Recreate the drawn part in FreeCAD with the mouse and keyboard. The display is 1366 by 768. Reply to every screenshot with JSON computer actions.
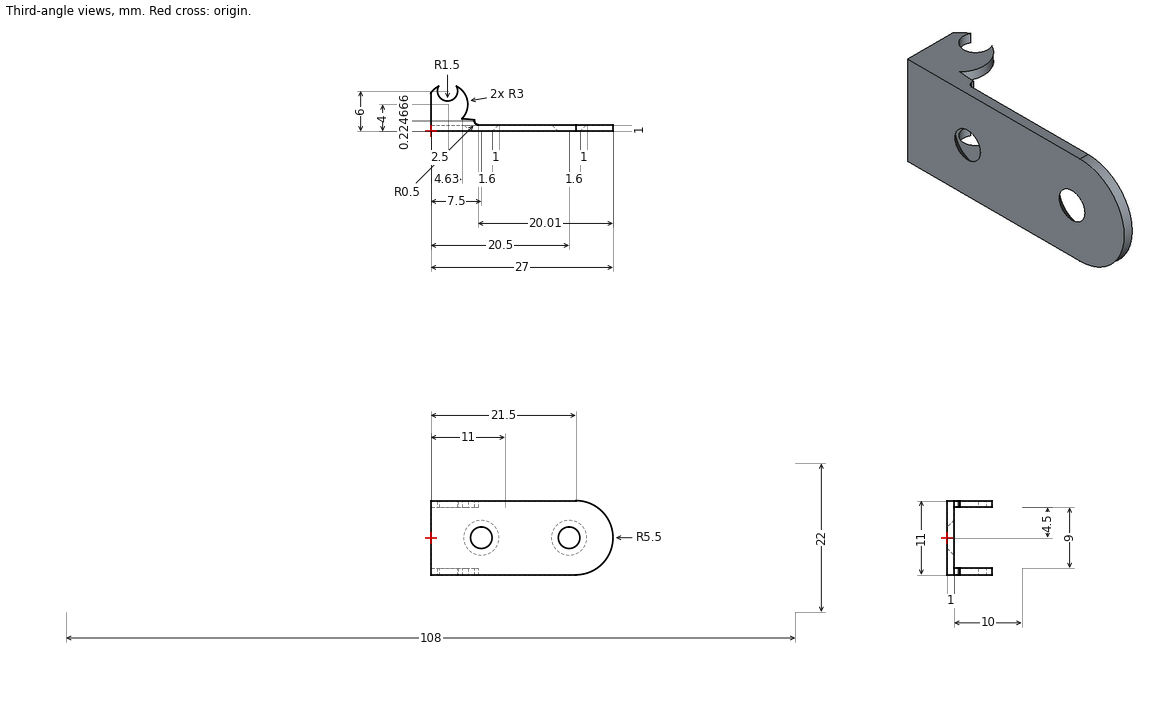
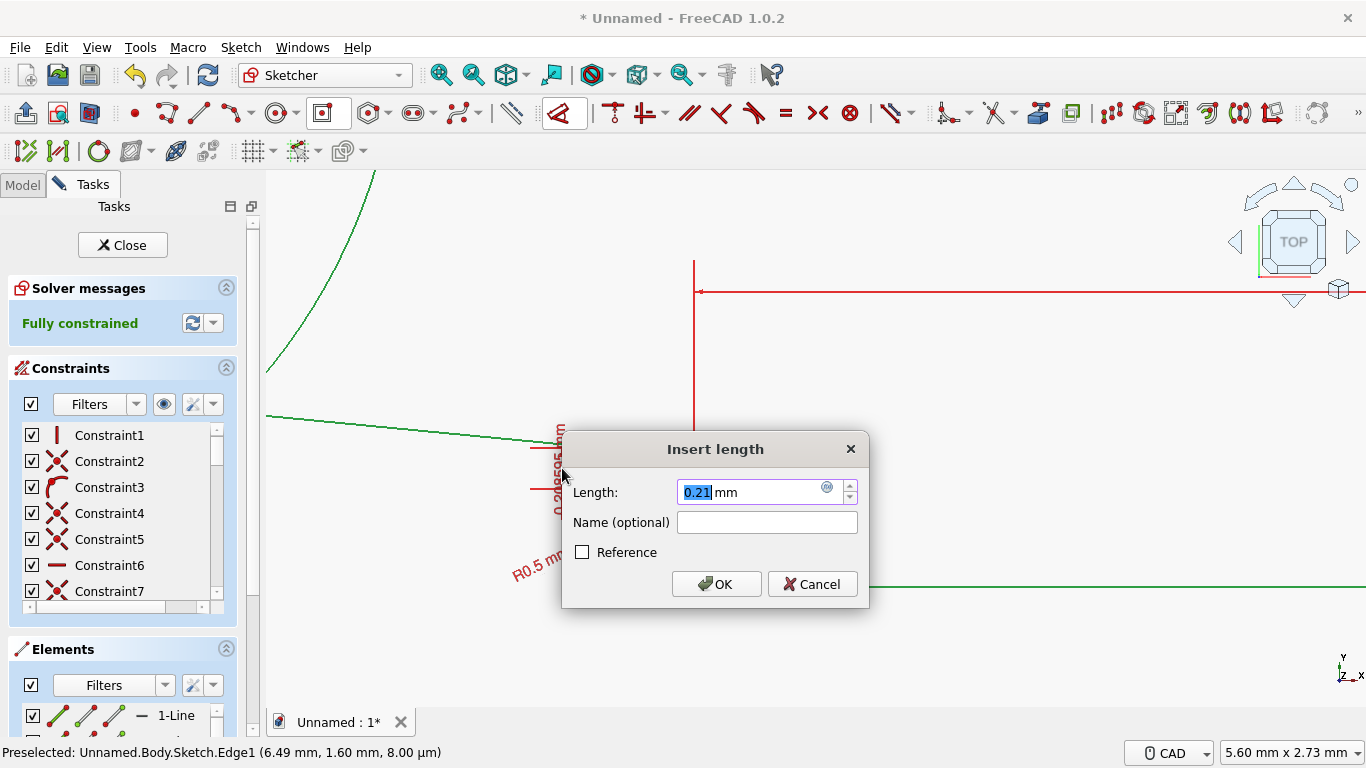
{"action": "type", "text": "0.224666"}
{"action": "key", "text": "Return"}
{"action": "key", "text": "Escape"}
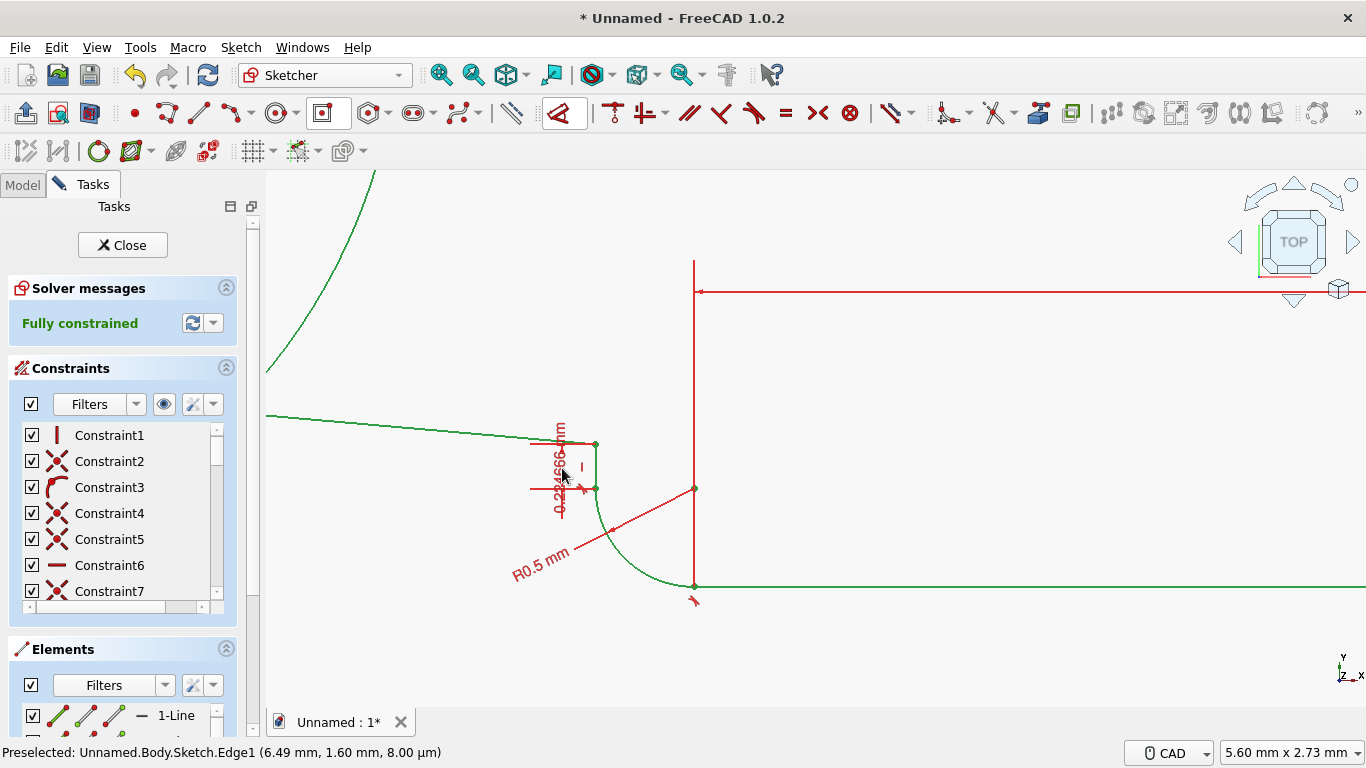
{"action": "left_click", "coordinate": [123, 245]}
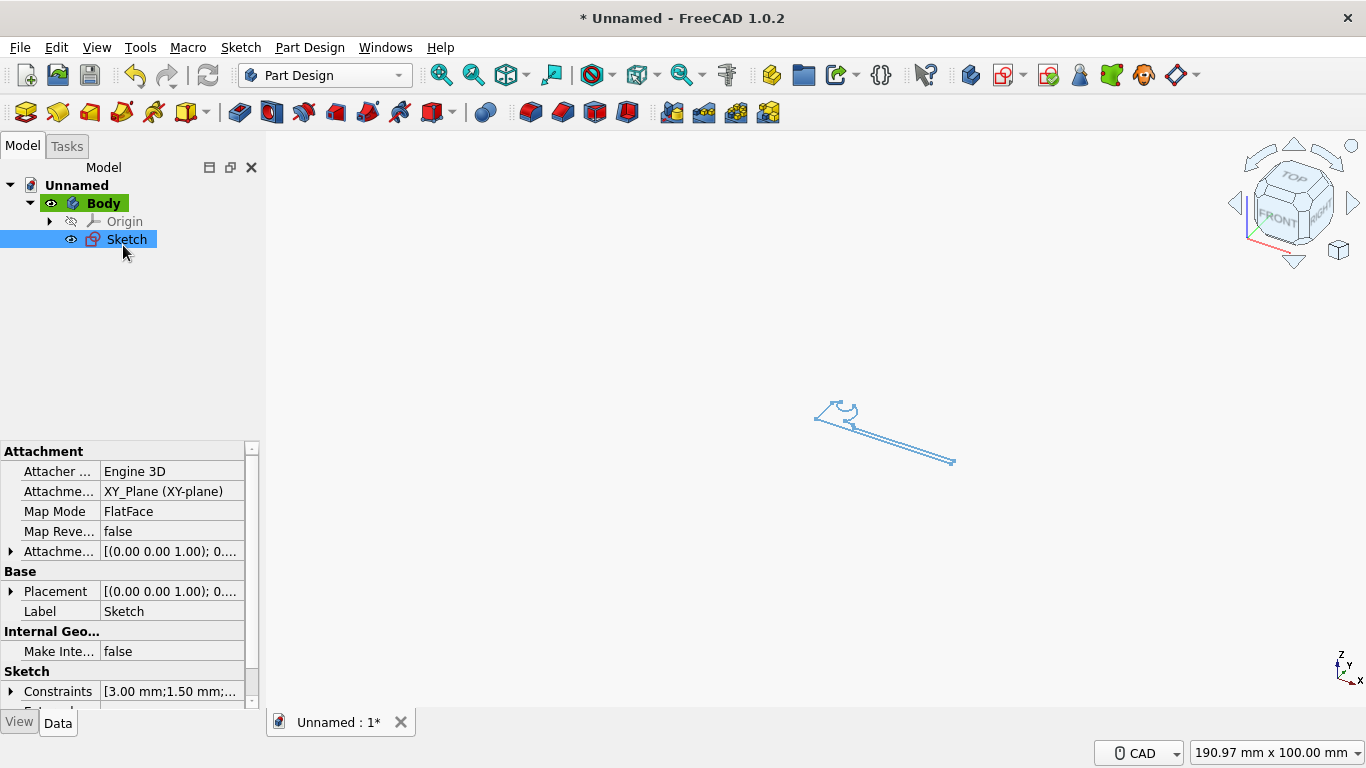
{"action": "left_click", "coordinate": [26, 112]}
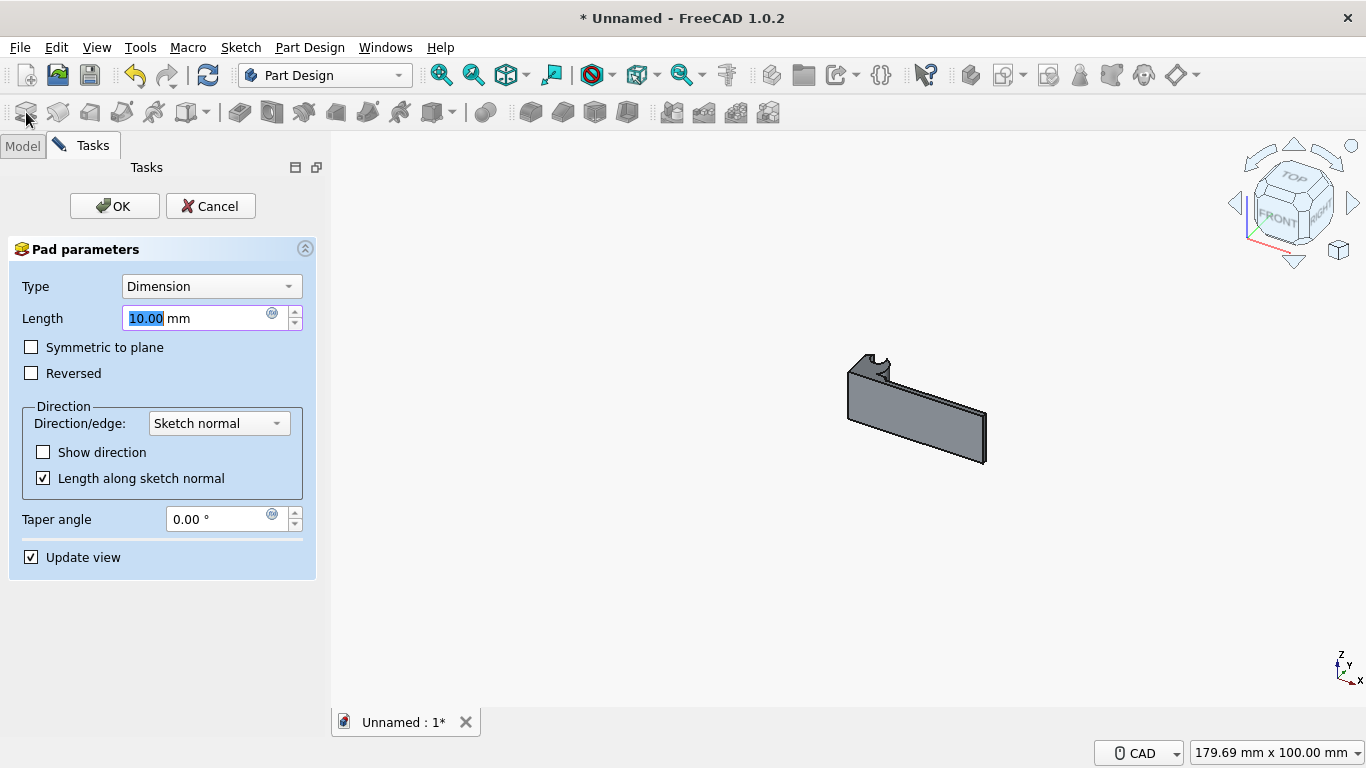
{"action": "type", "text": "11"}
{"action": "key", "text": "Tab"}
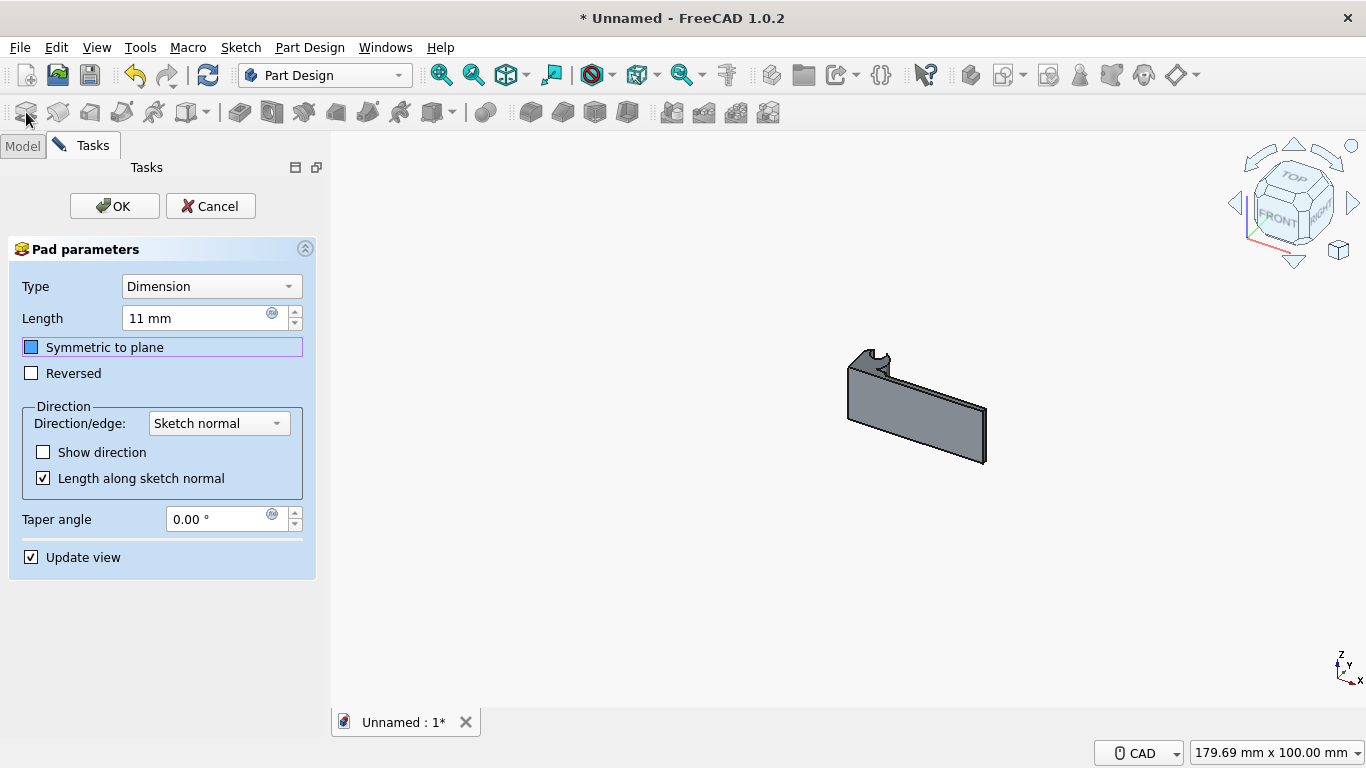
{"action": "left_click", "coordinate": [30, 347]}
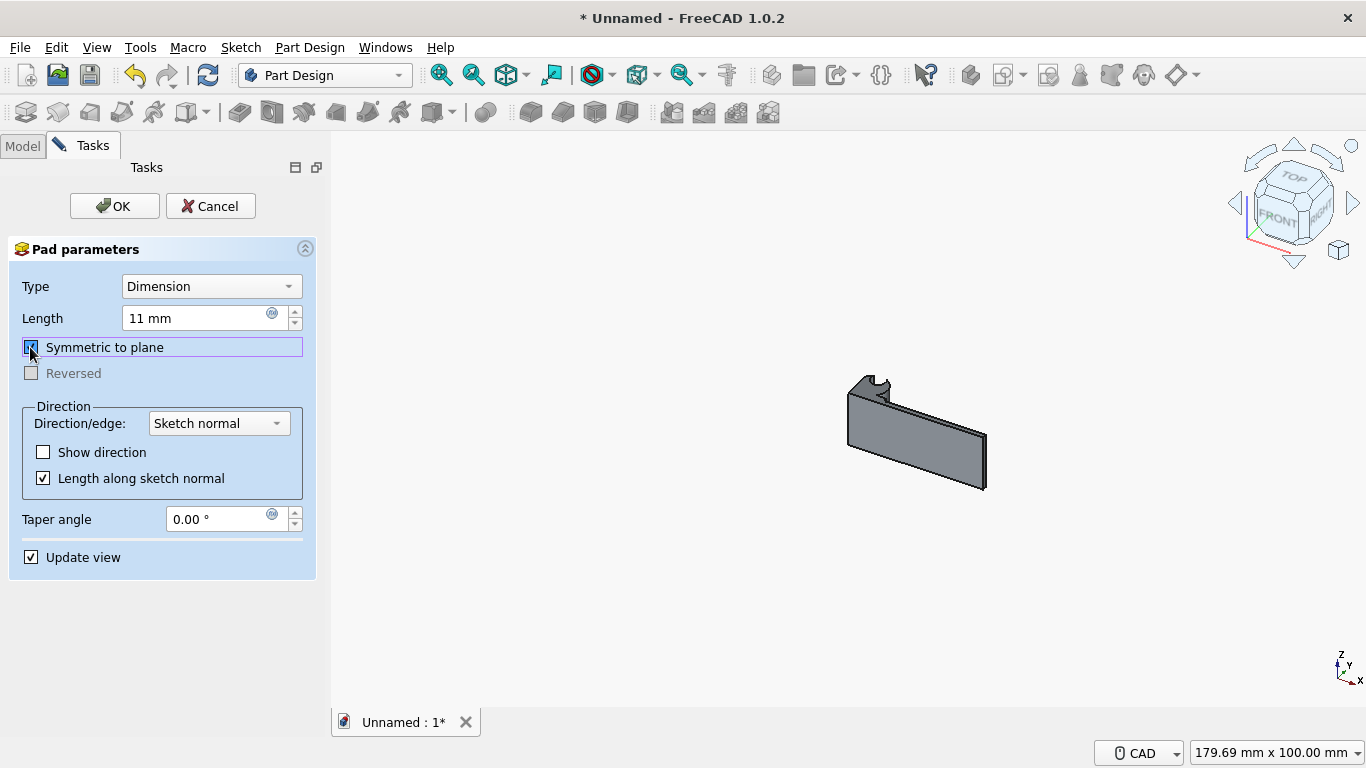
{"action": "left_click", "coordinate": [115, 206]}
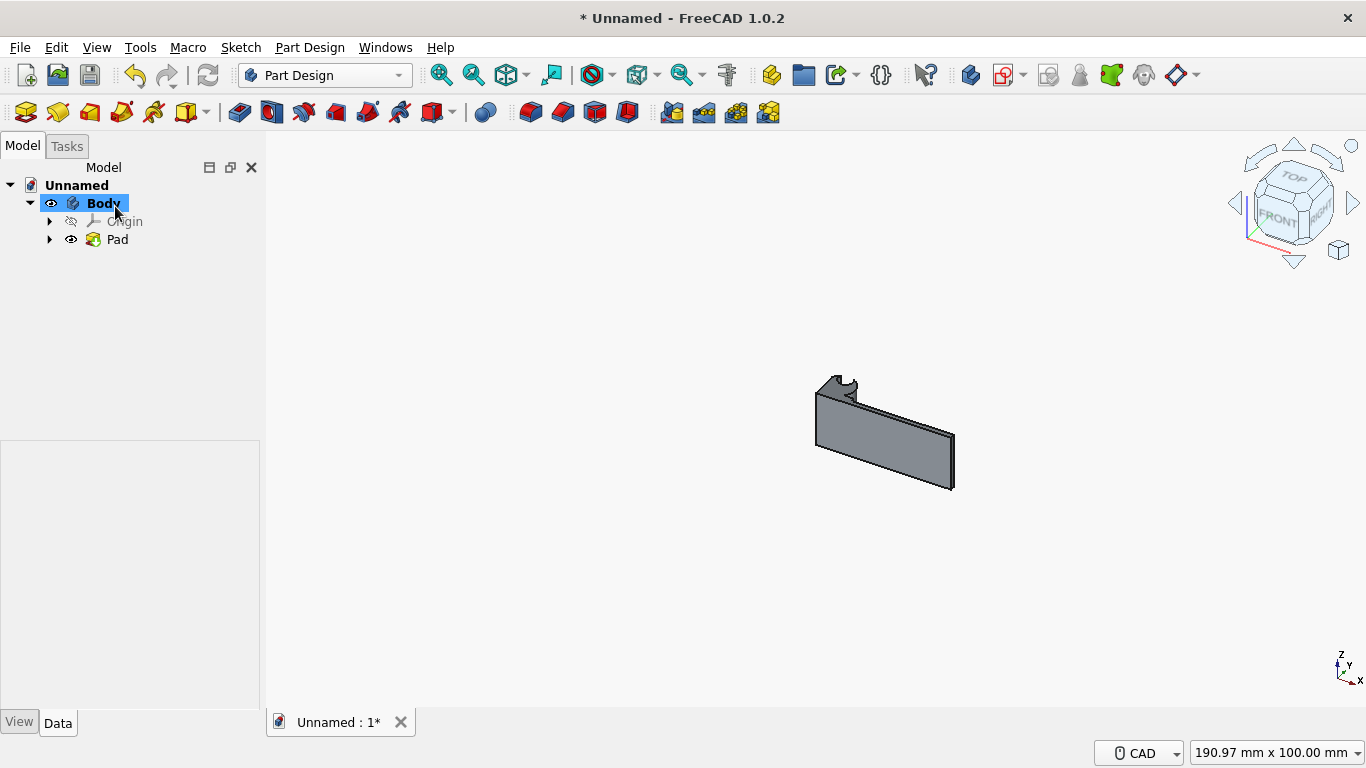
{"action": "left_click", "coordinate": [442, 76]}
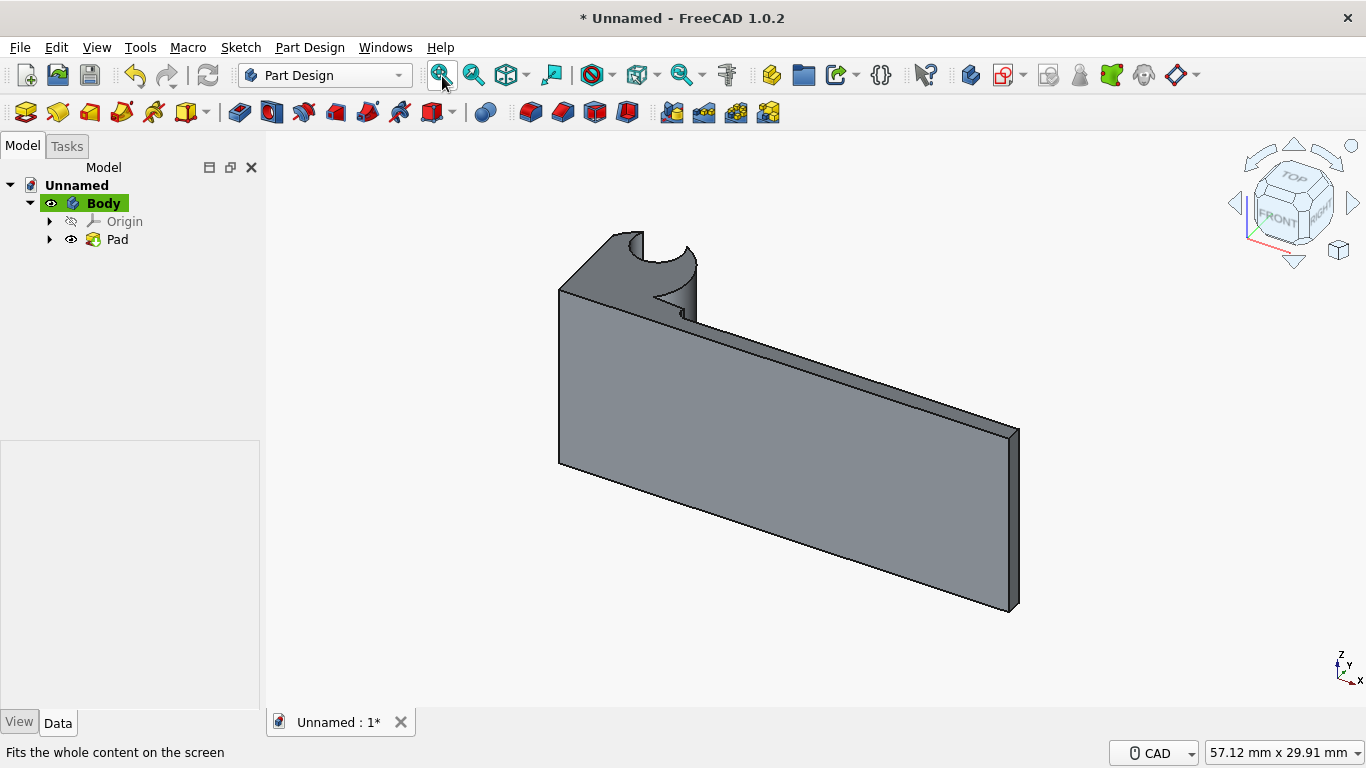
{"action": "left_click", "coordinate": [1004, 76]}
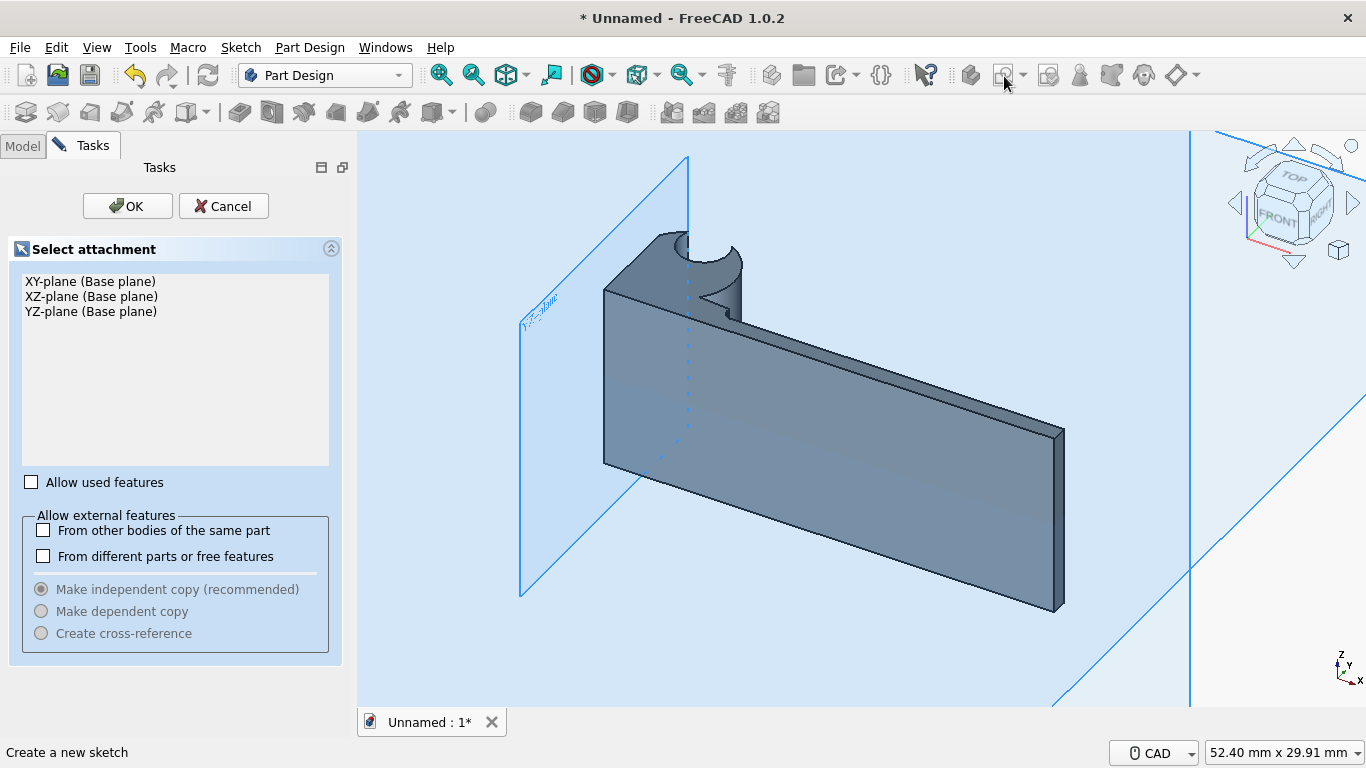
{"action": "left_click", "coordinate": [82, 296]}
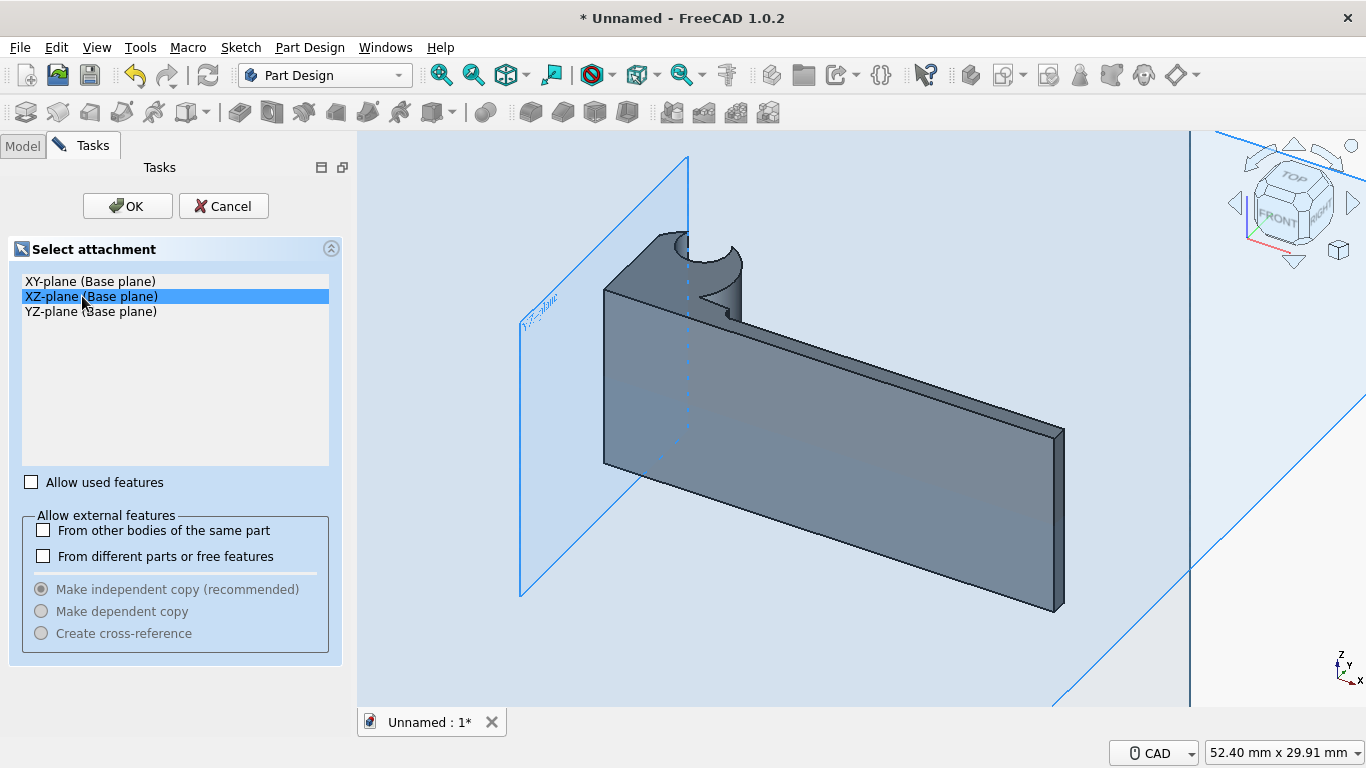
{"action": "left_click", "coordinate": [128, 206]}